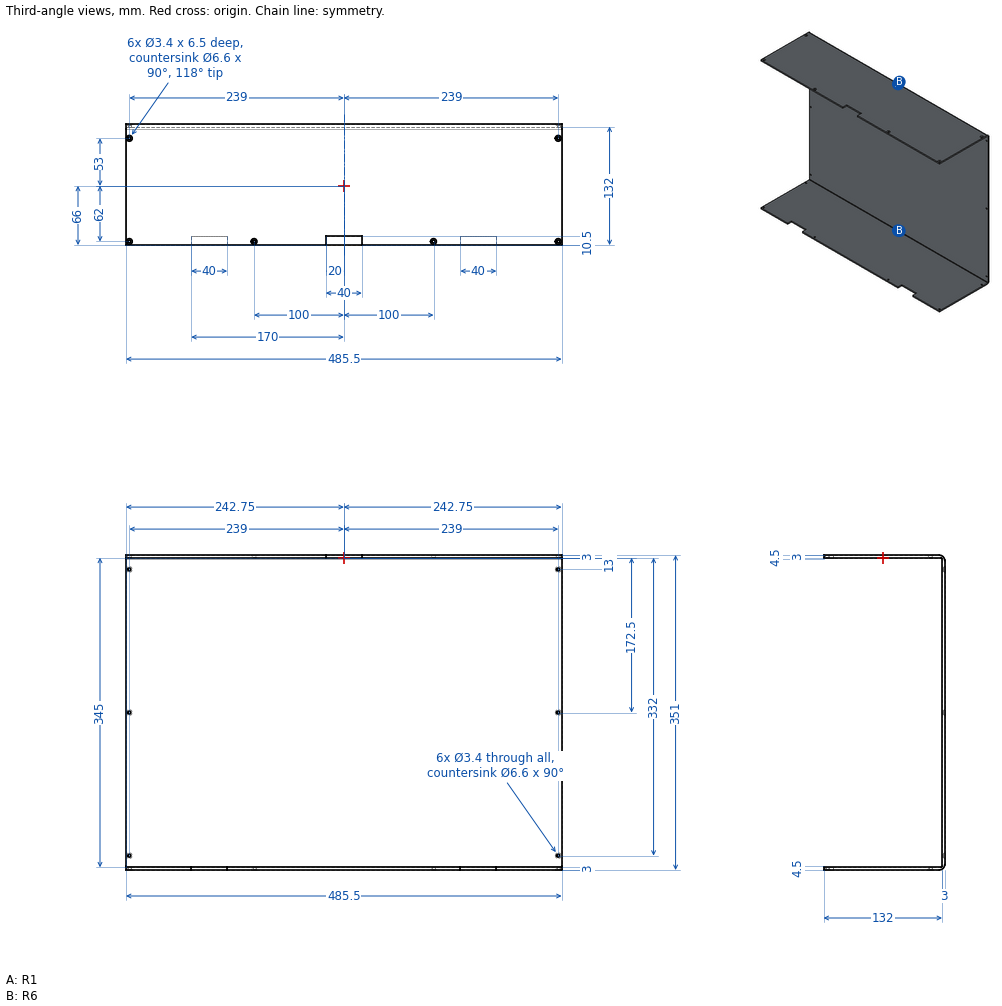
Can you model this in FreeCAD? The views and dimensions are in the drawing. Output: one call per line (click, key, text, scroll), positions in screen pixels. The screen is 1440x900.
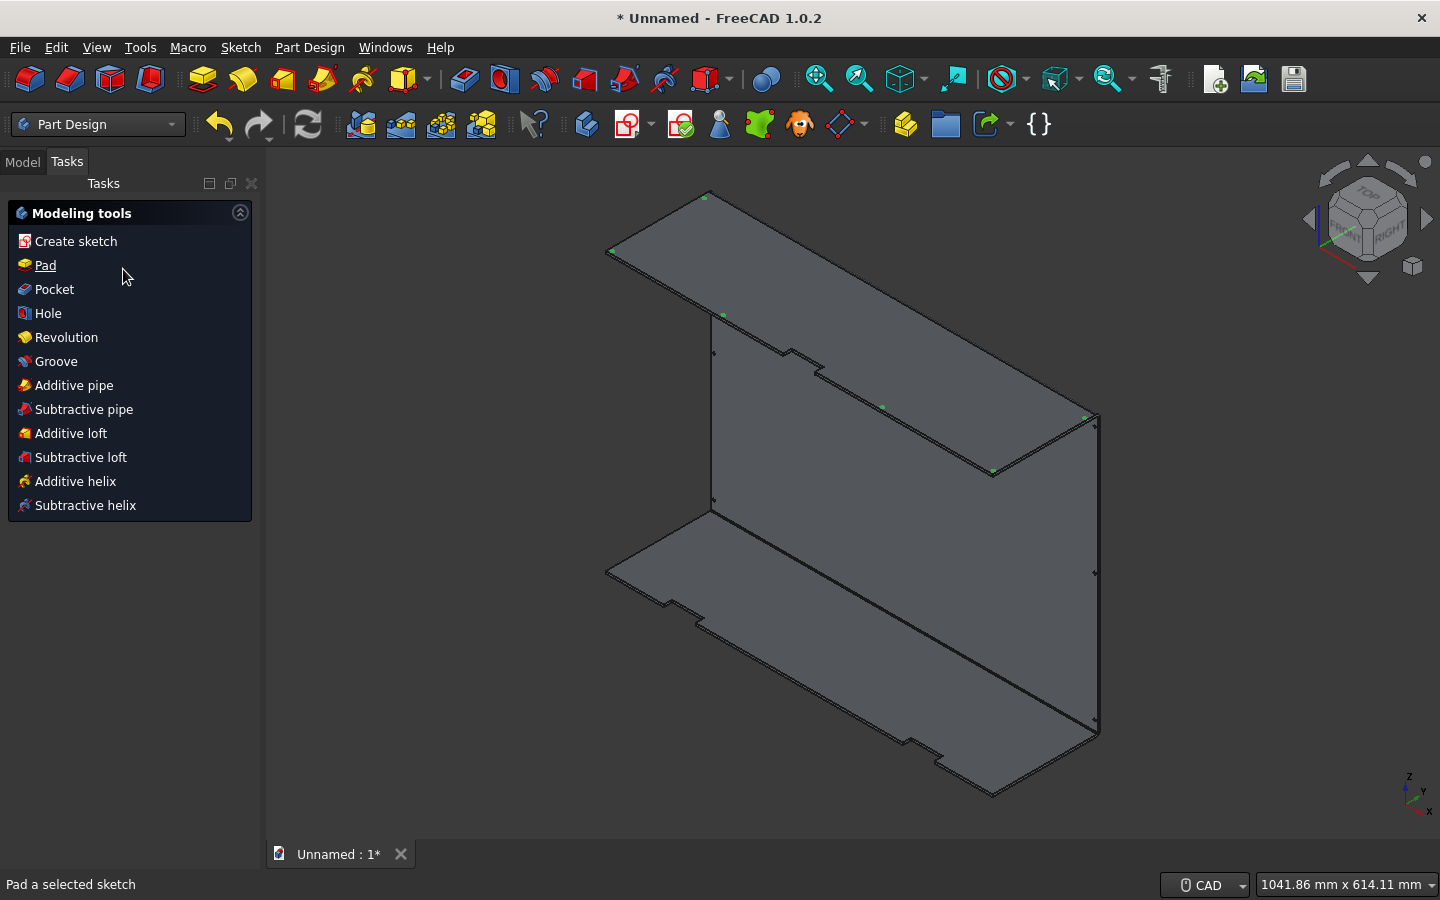
click(506, 80)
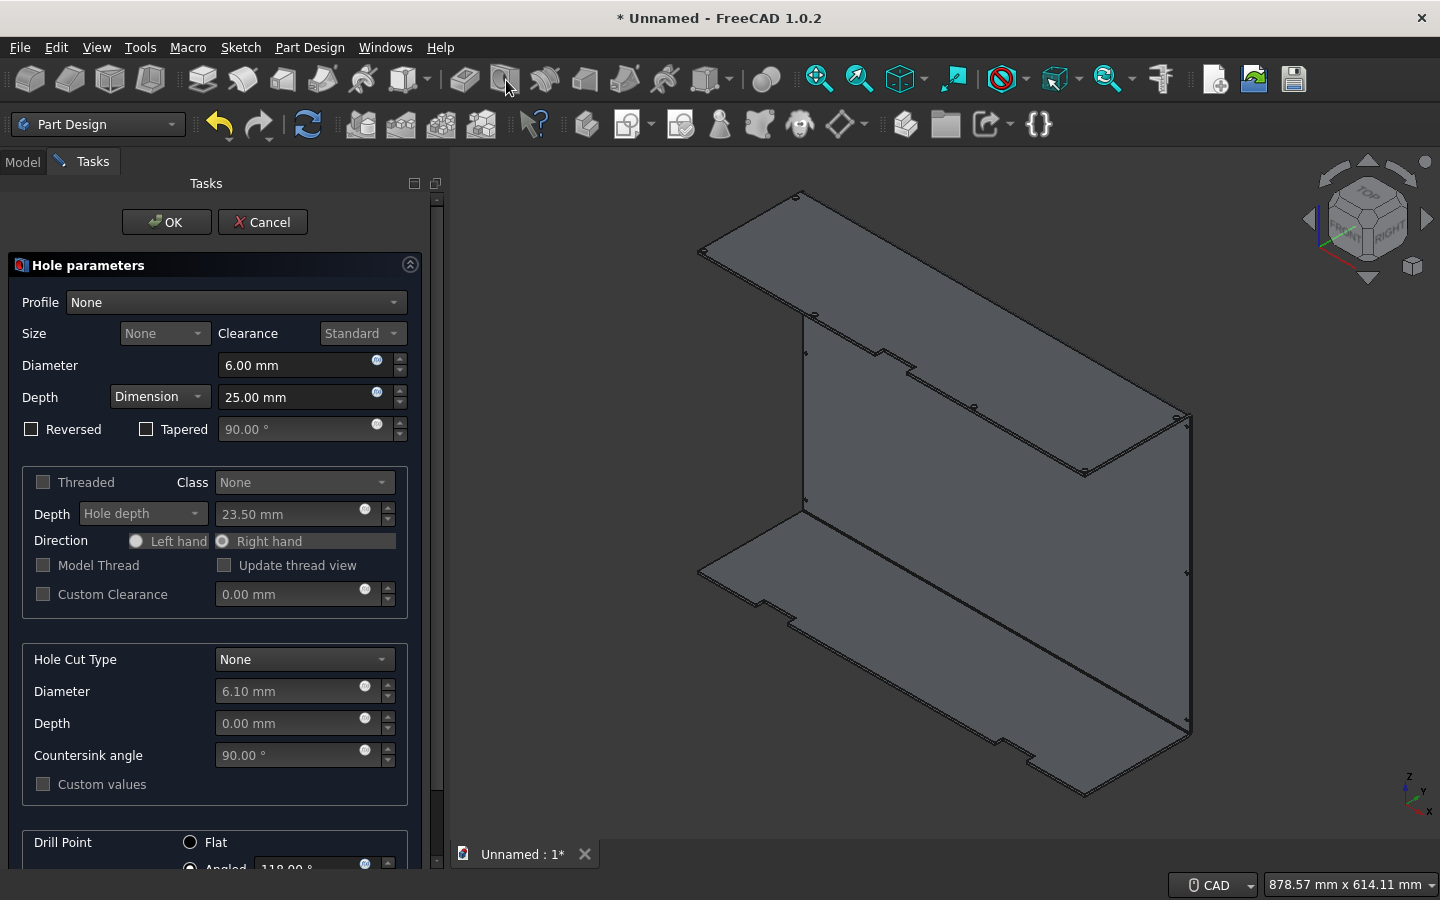
triple_click(305, 365)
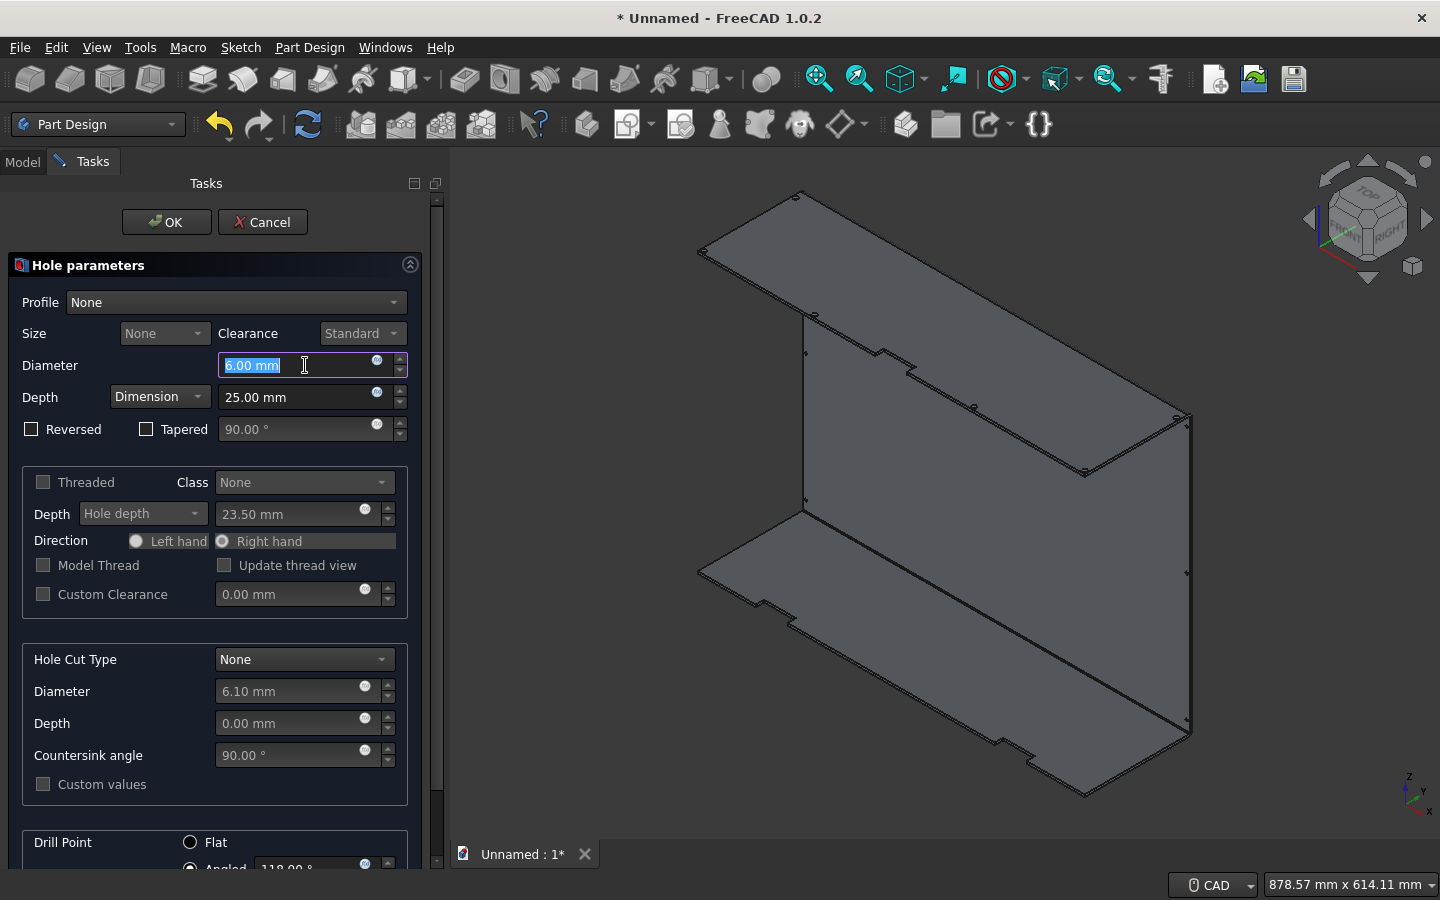
text(3.4)
key(Tab)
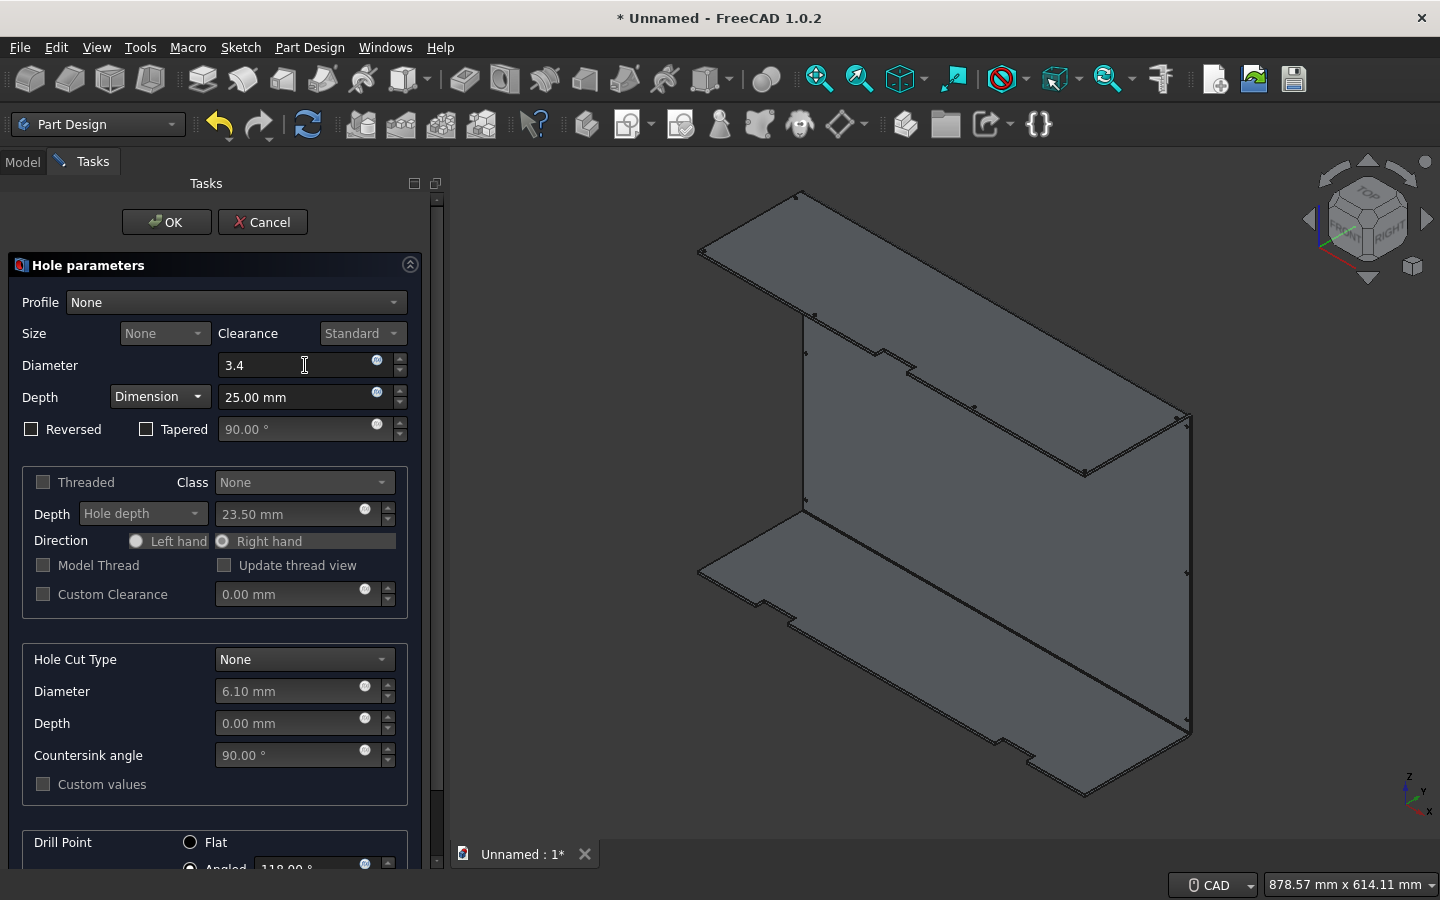
triple_click(305, 397)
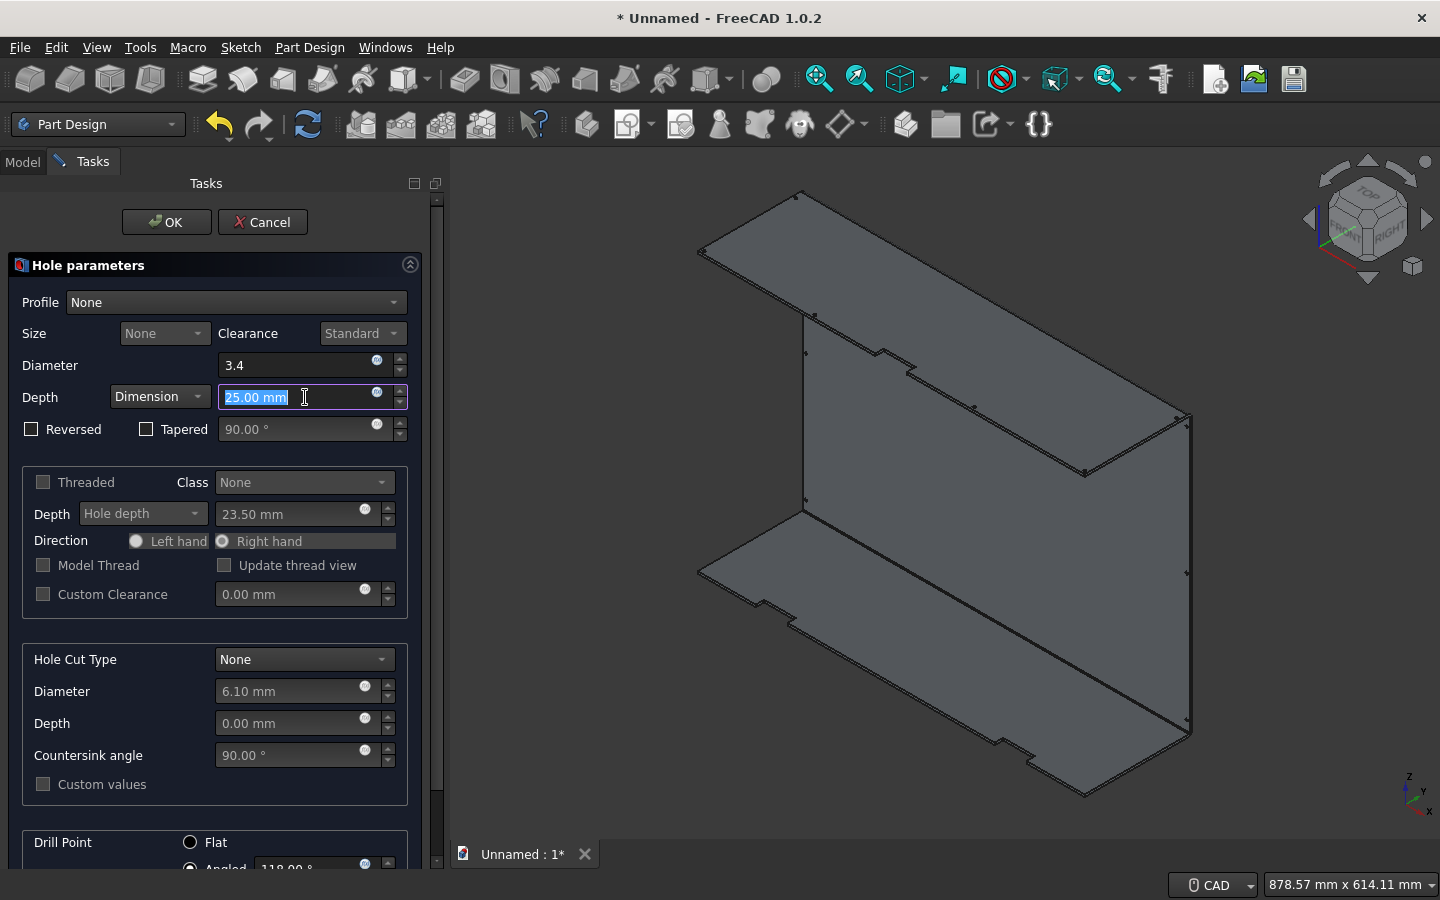
text(6.5)
key(Tab)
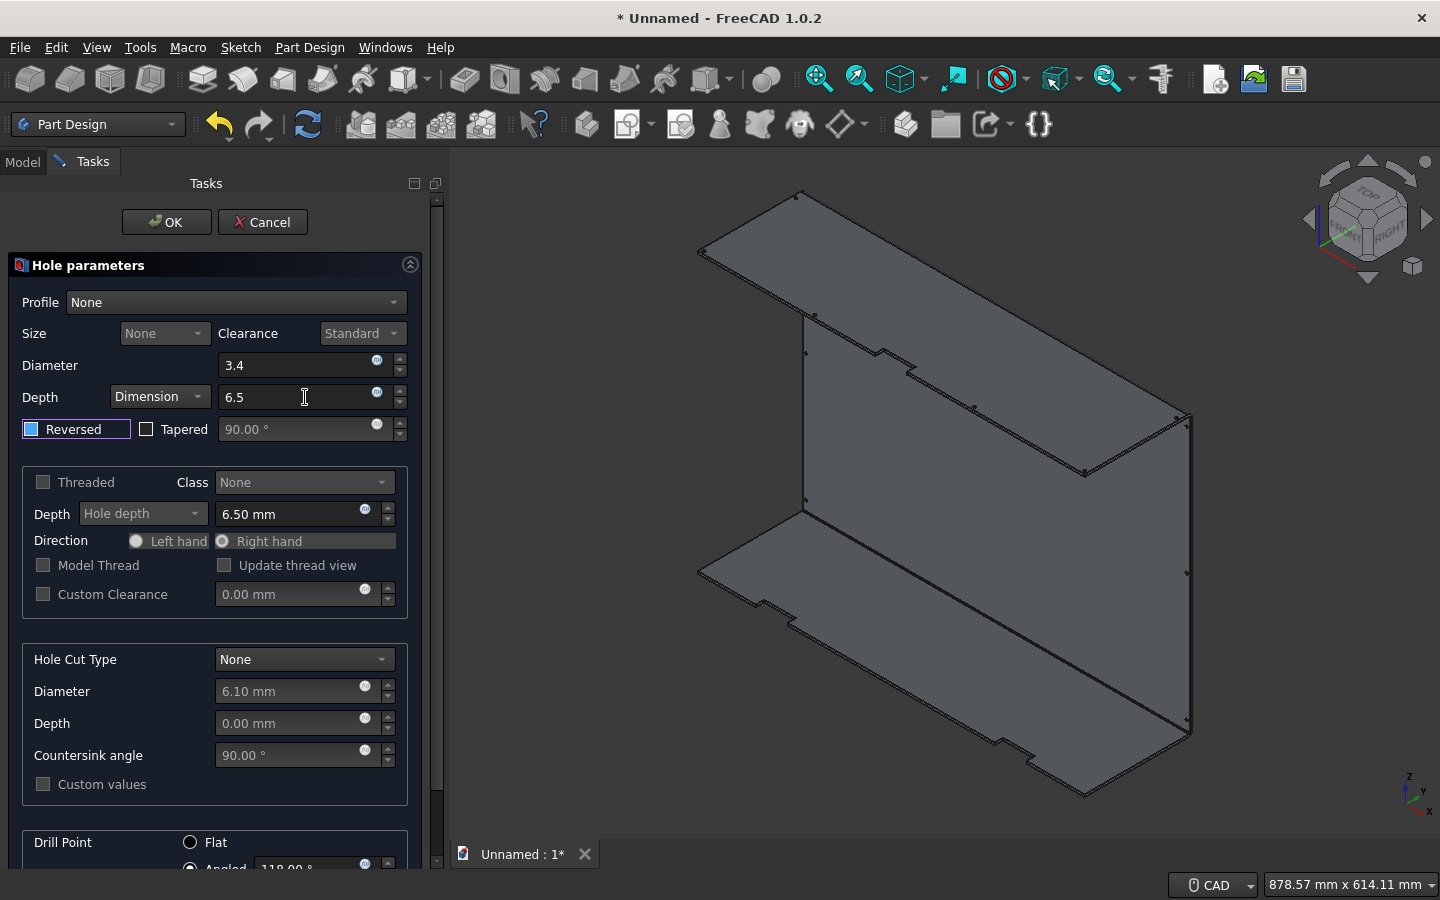
click(306, 660)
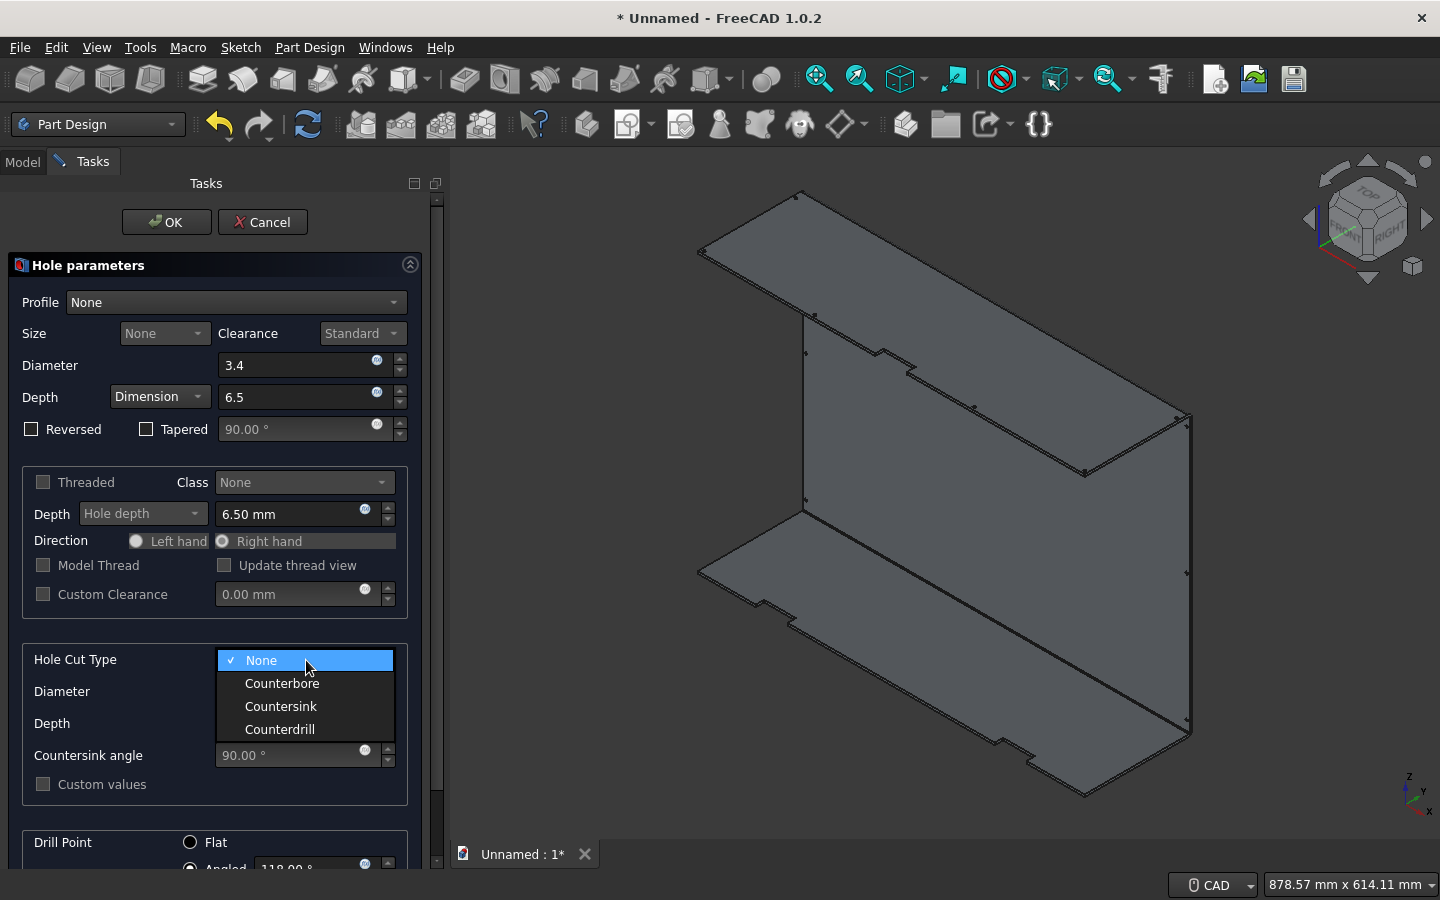
click(304, 706)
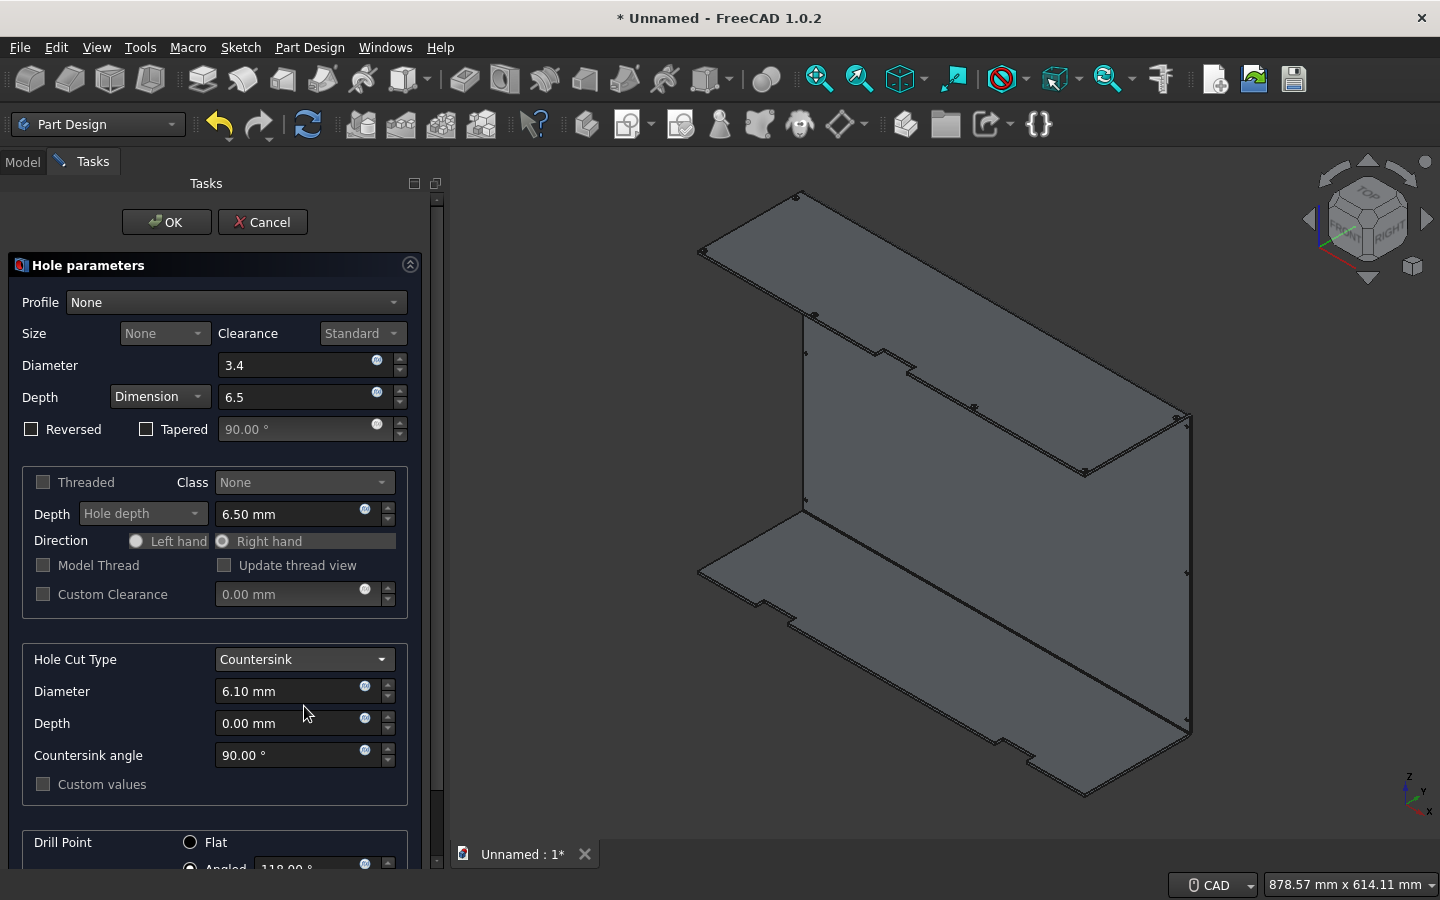
triple_click(298, 691)